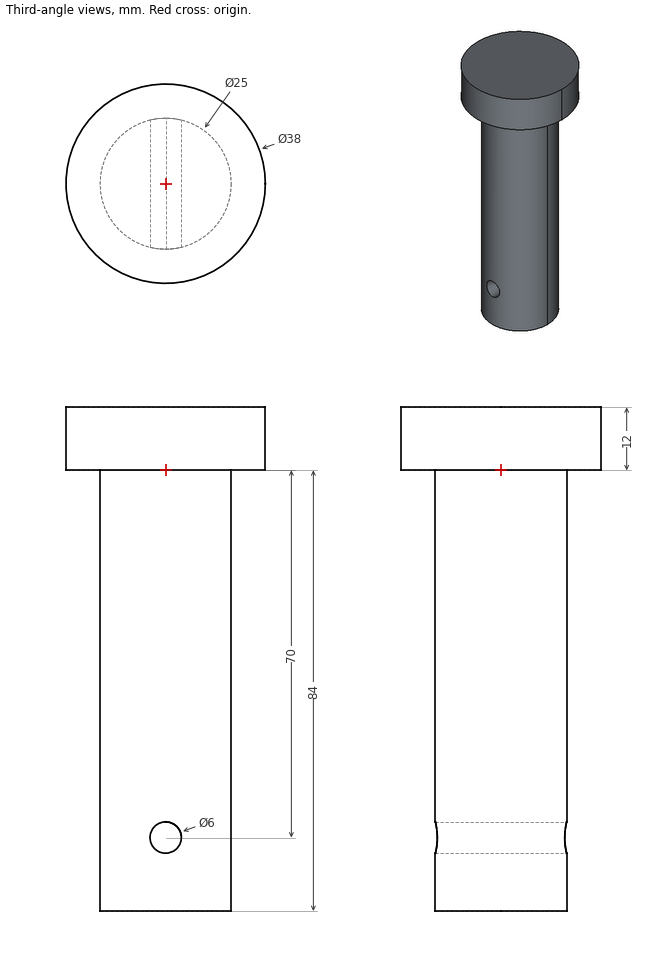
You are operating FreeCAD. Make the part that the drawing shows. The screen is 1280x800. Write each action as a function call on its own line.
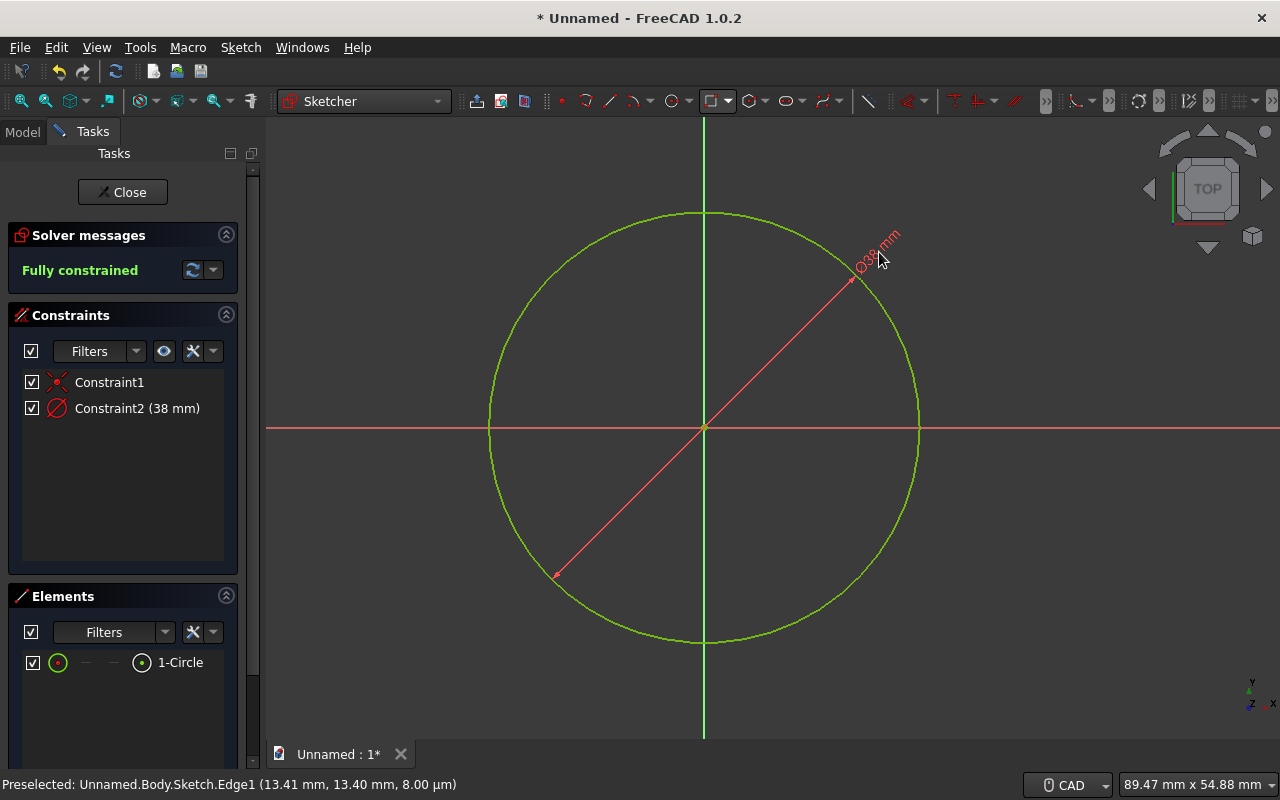
click(123, 192)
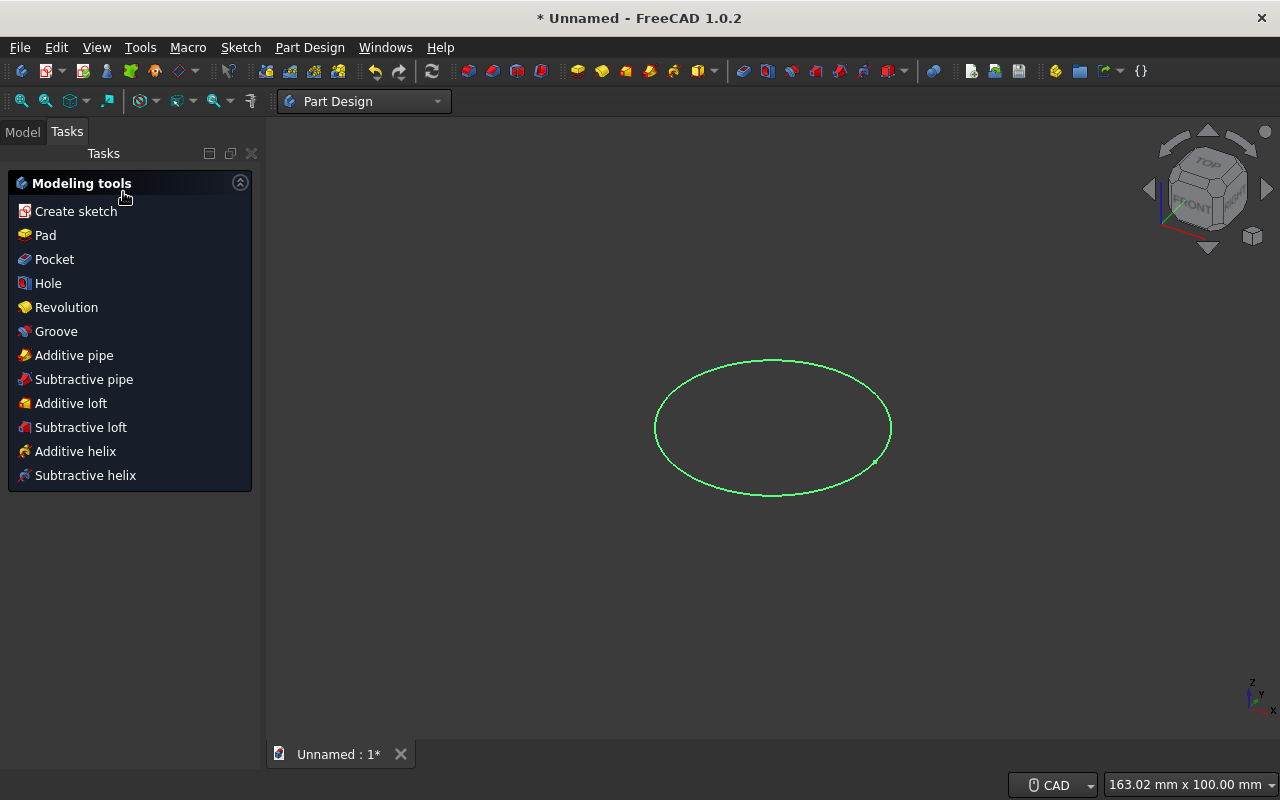
click(578, 72)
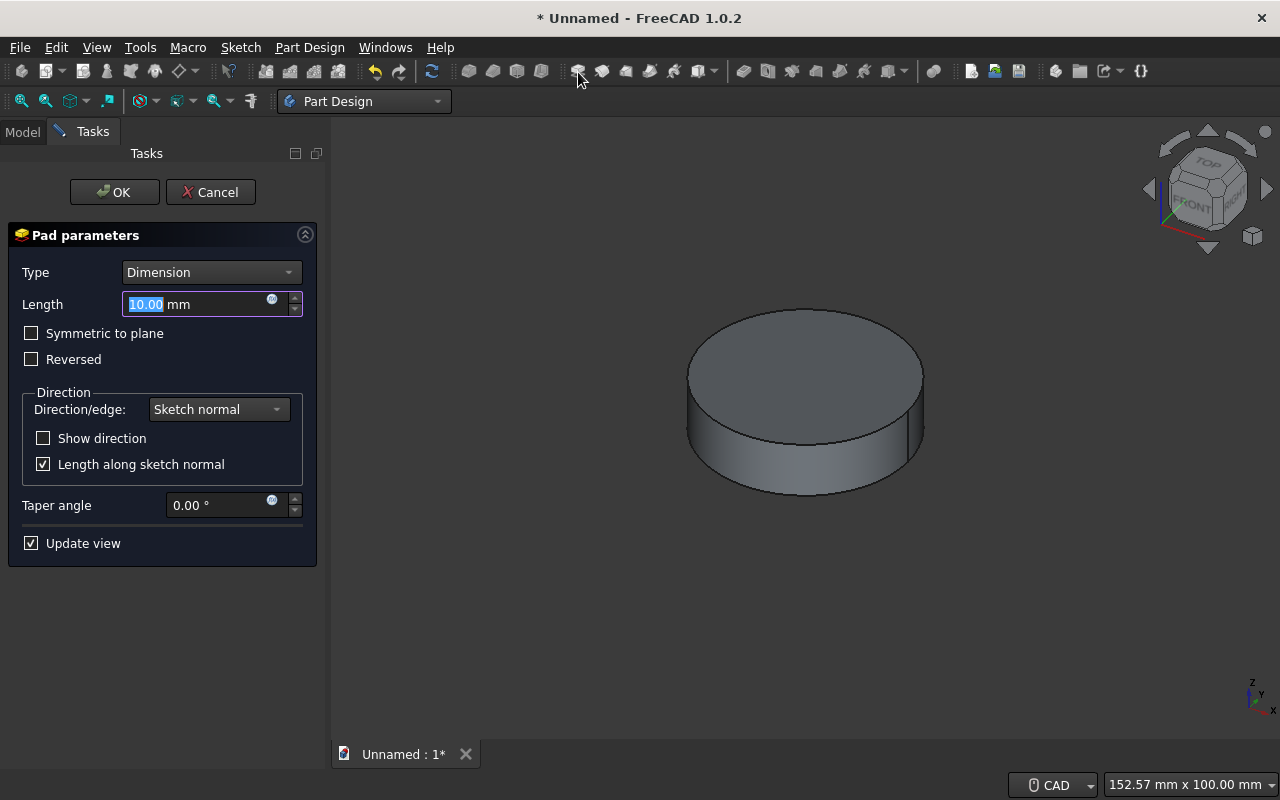
text(12)
key(Tab)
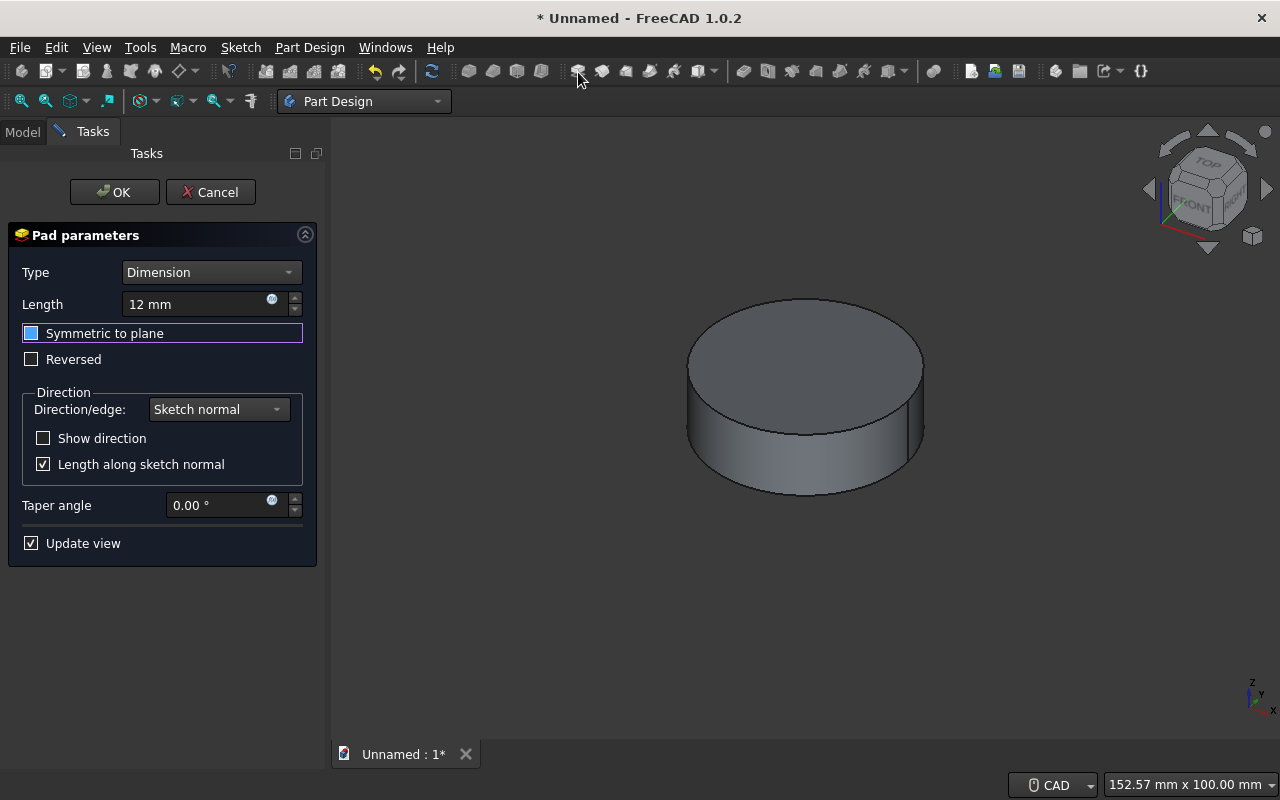
click(115, 192)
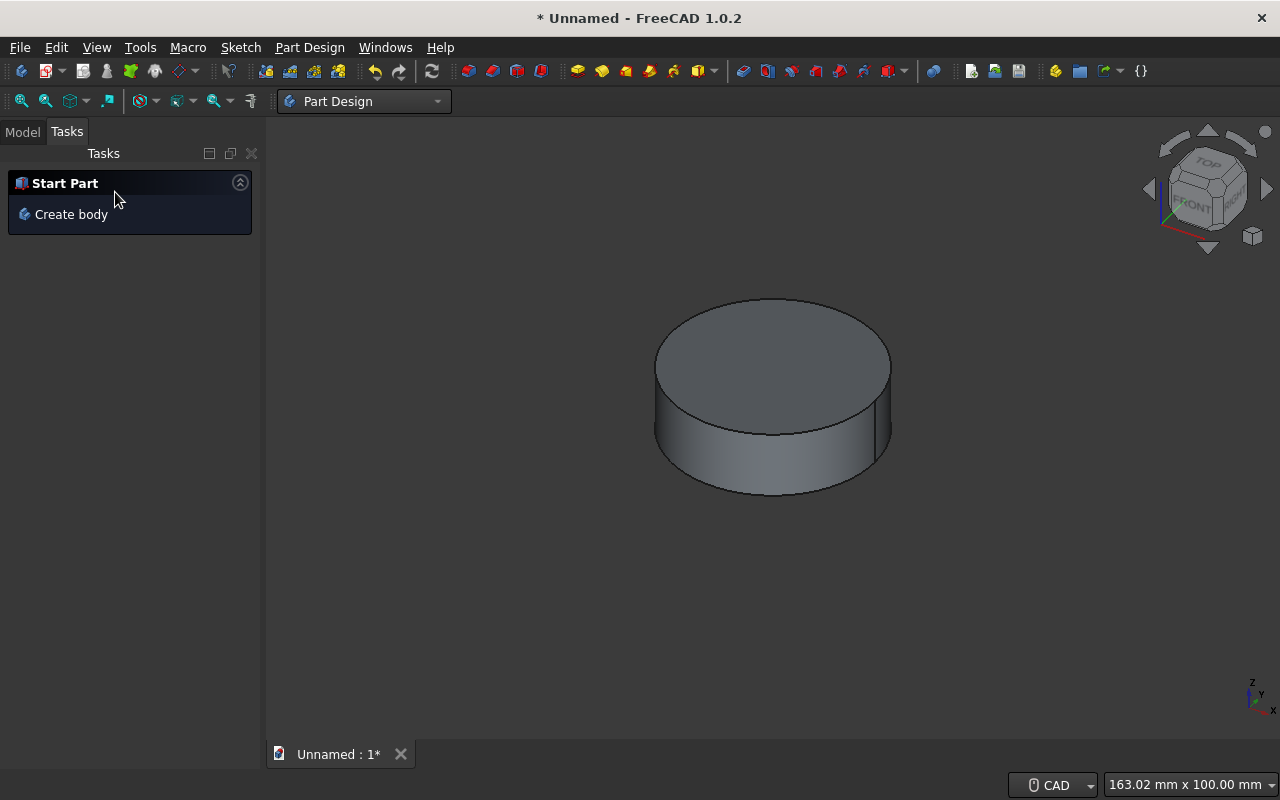
click(22, 102)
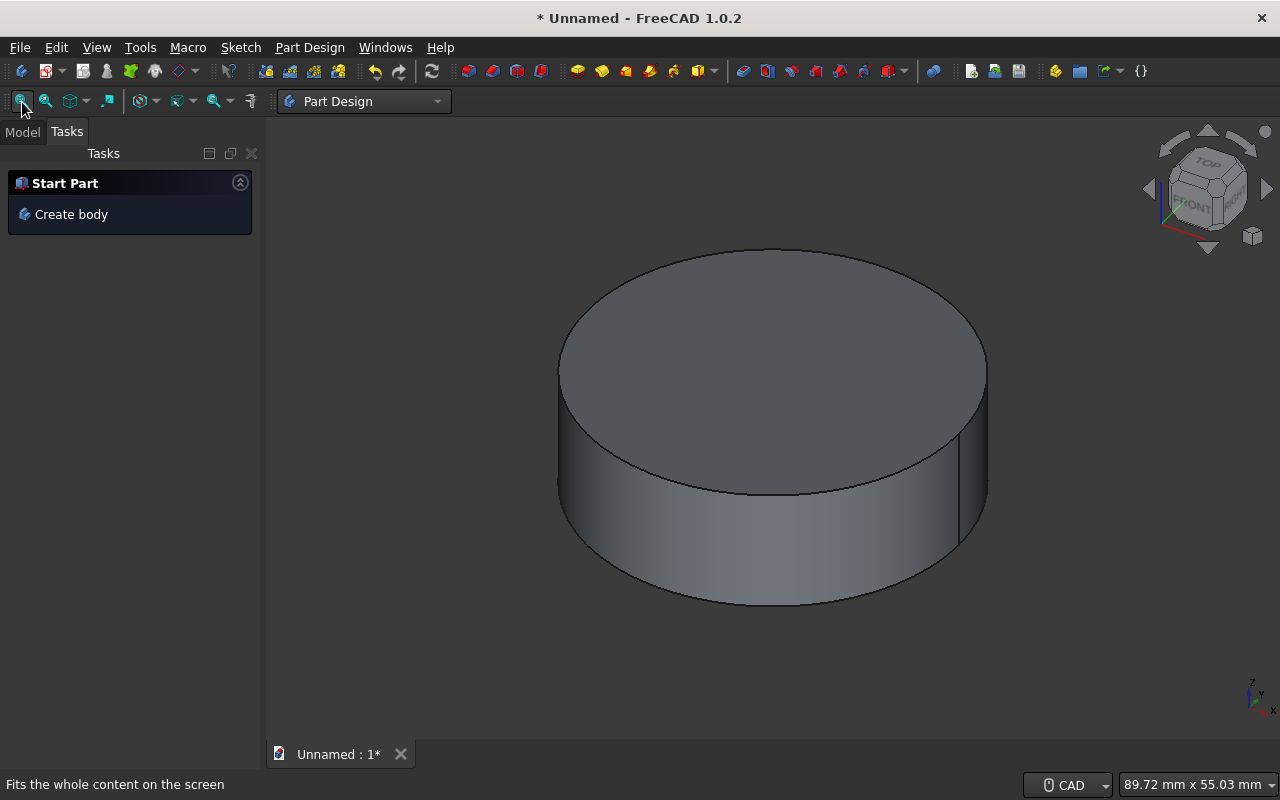
click(46, 72)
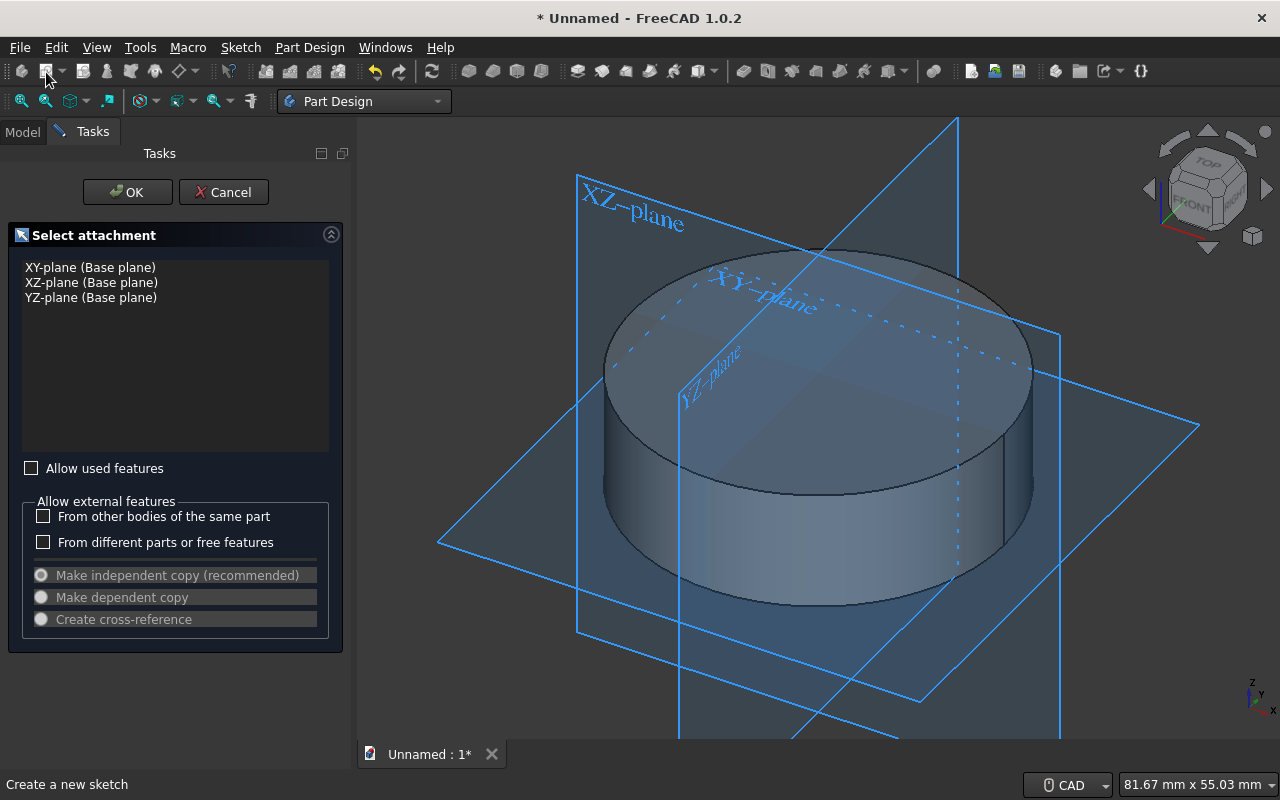
click(82, 268)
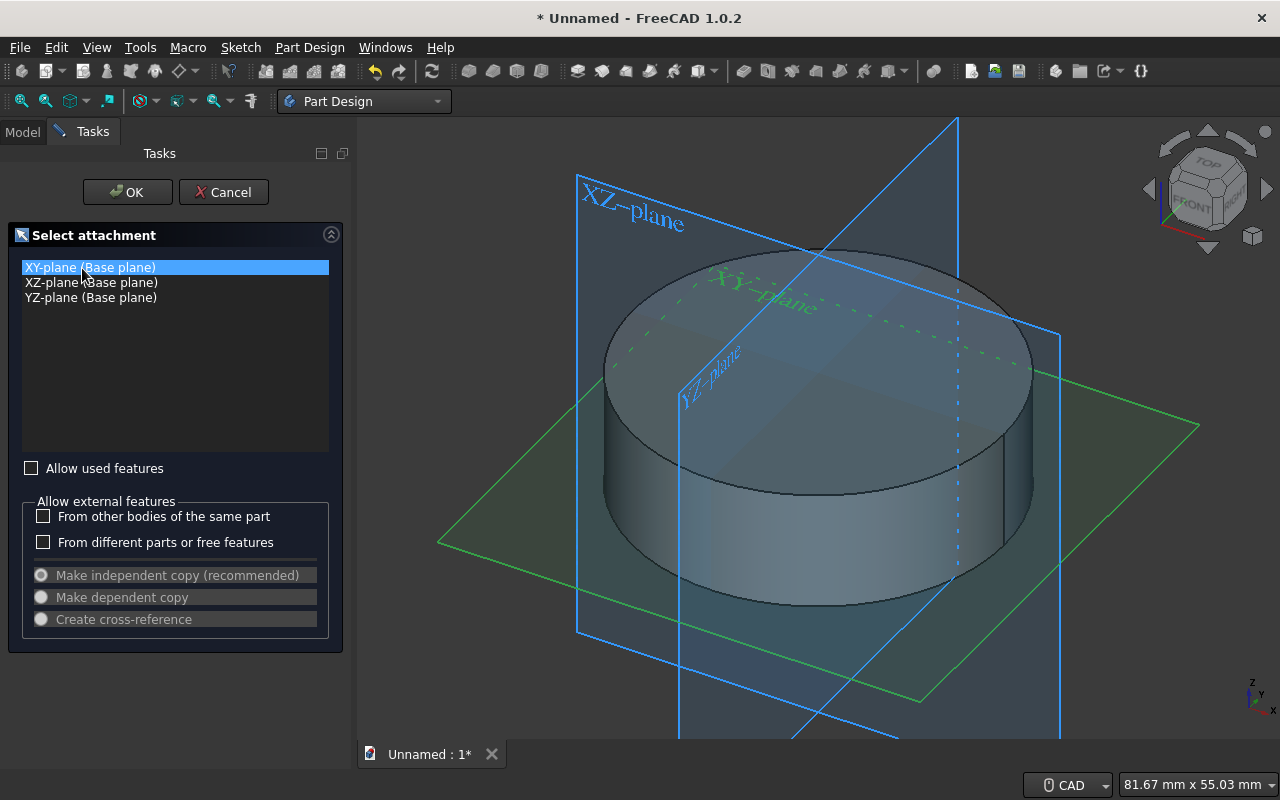
click(128, 192)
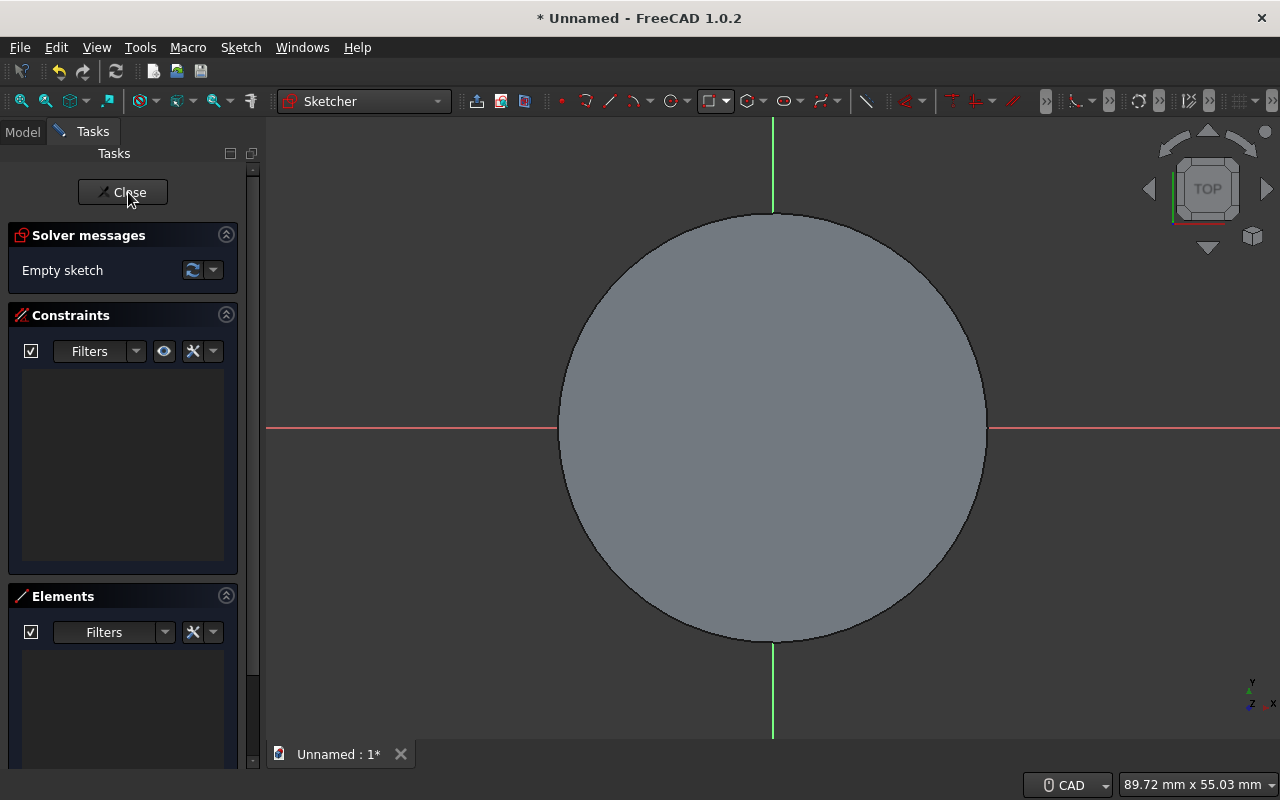
key(q)
key(s)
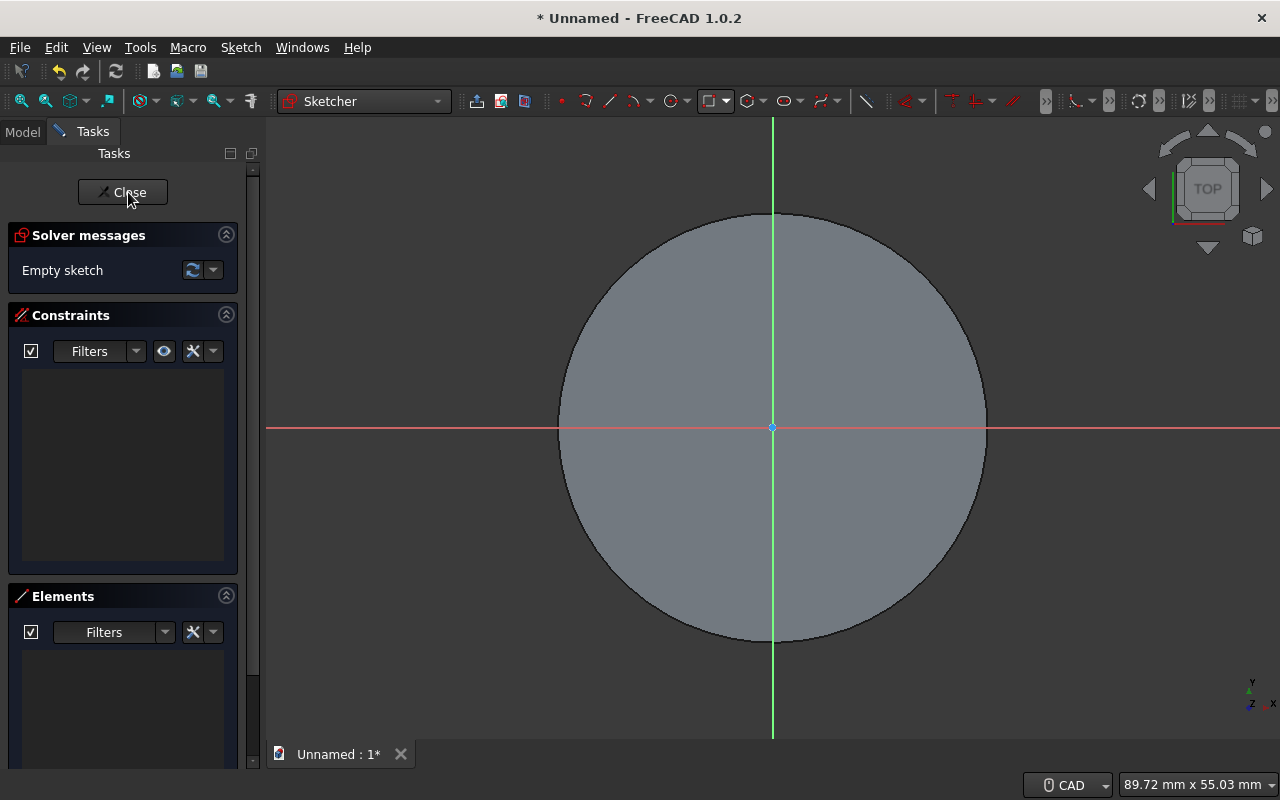
scroll(912, 428, up, 2)